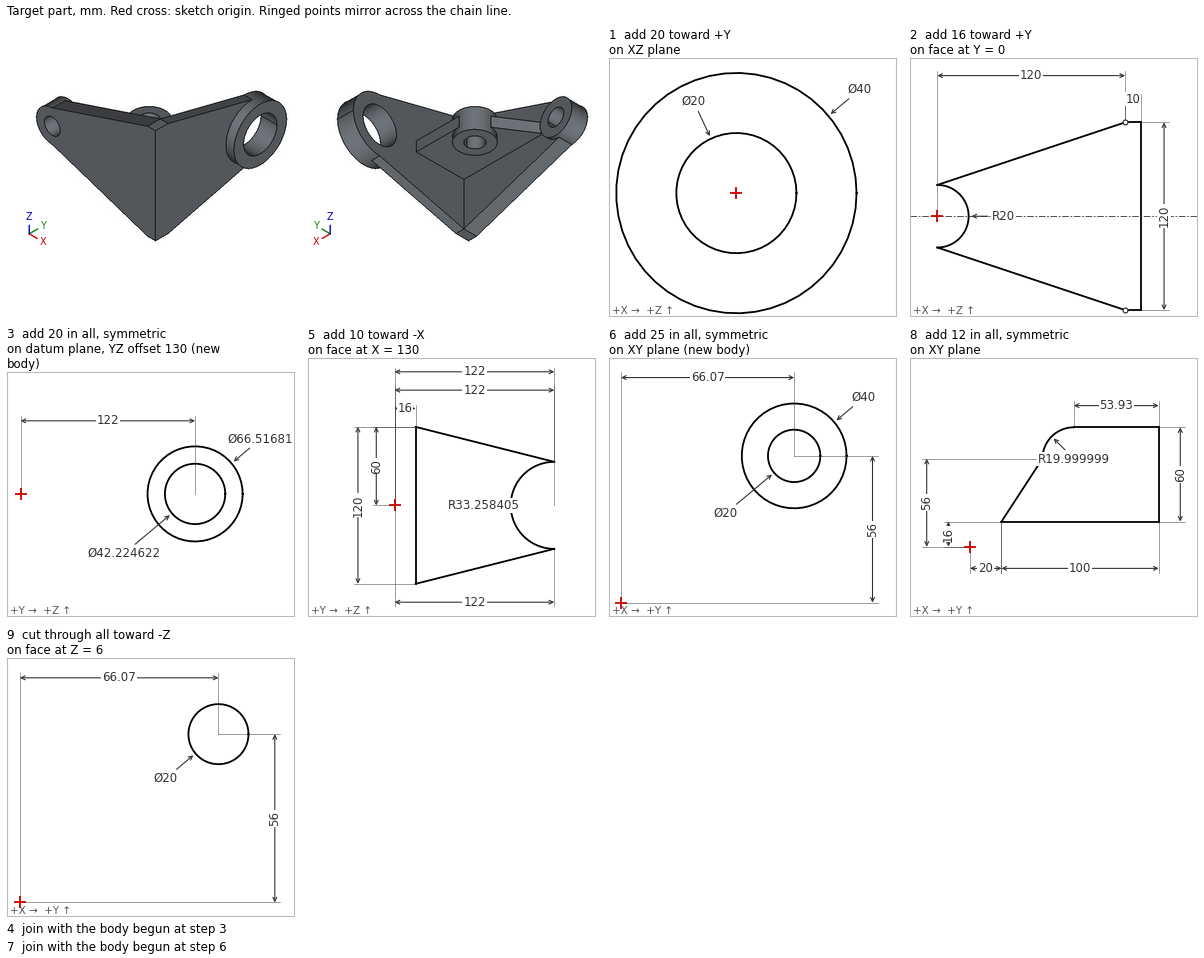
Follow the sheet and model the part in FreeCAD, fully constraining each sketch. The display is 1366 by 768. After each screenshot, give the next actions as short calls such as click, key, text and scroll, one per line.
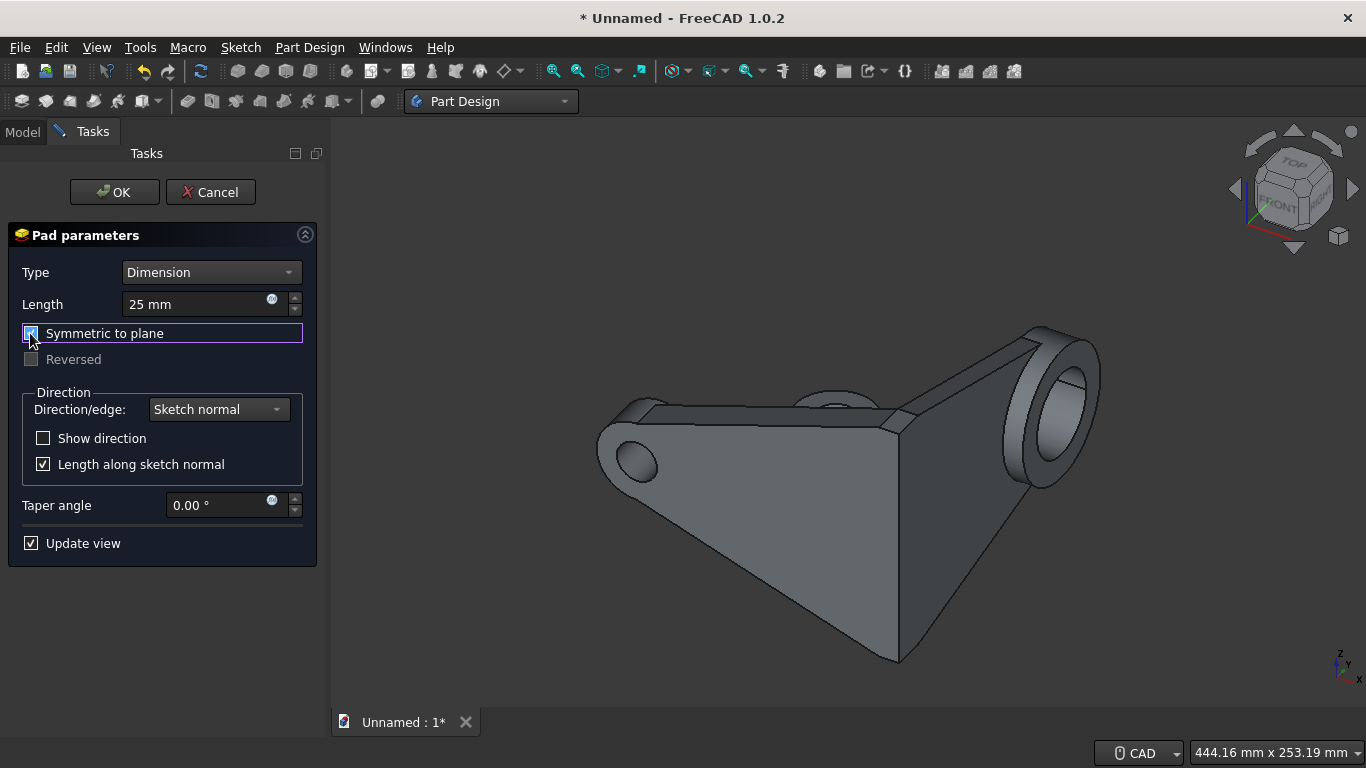
click(115, 192)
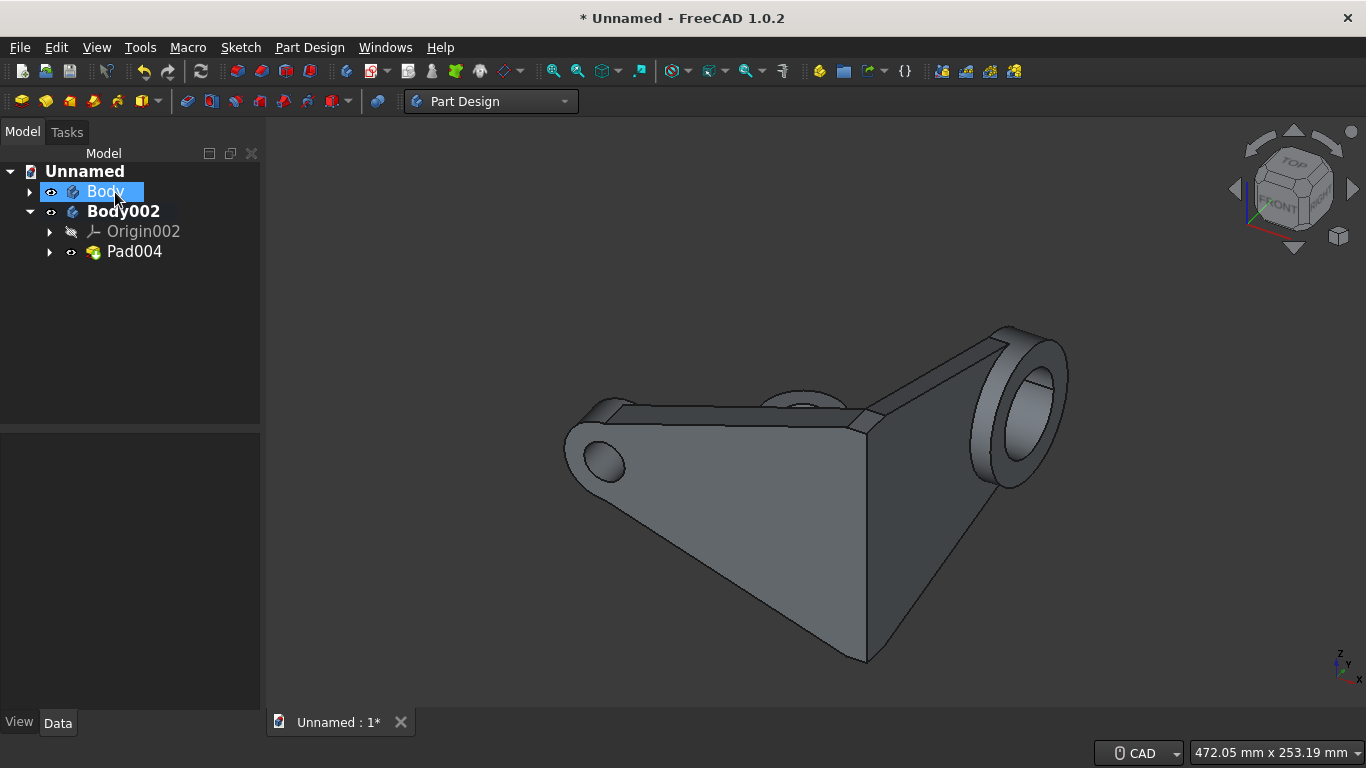
click(554, 72)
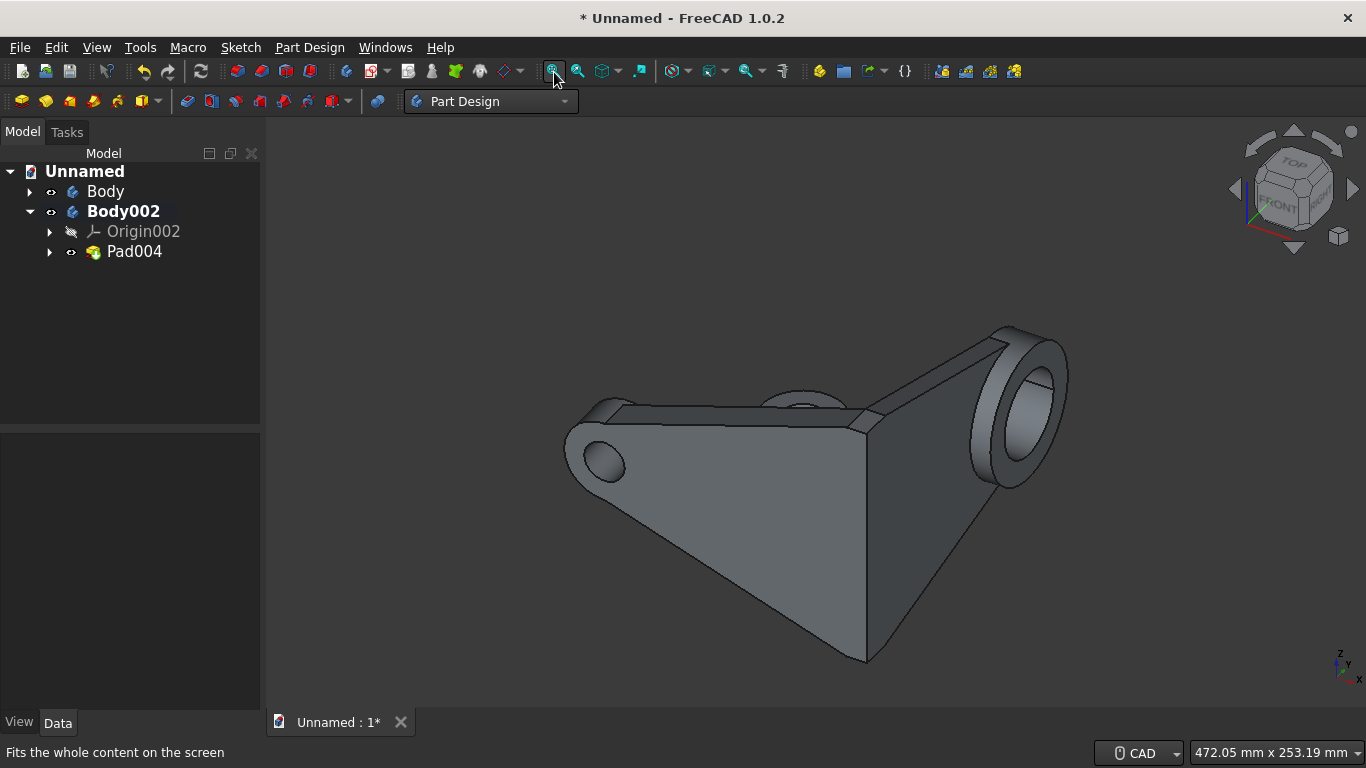
double_click(96, 192)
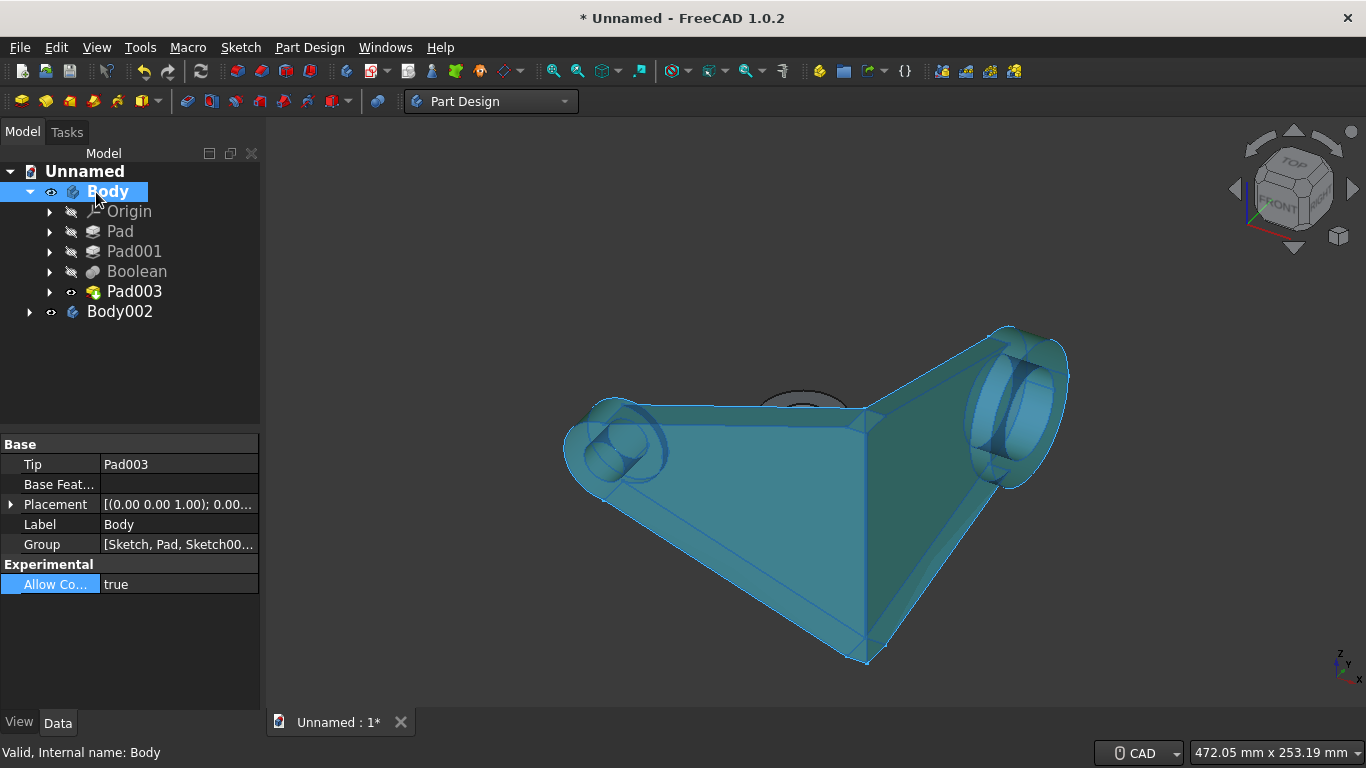
click(96, 312)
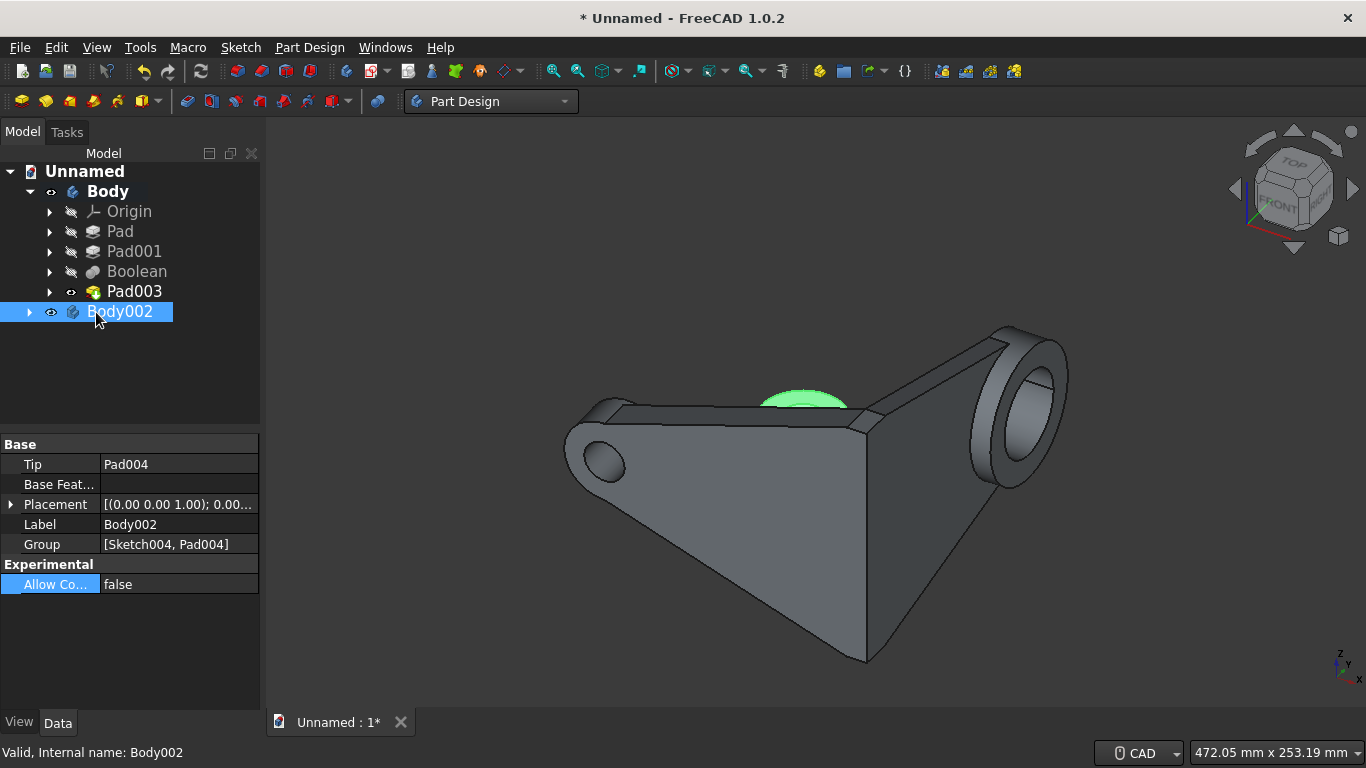
click(378, 102)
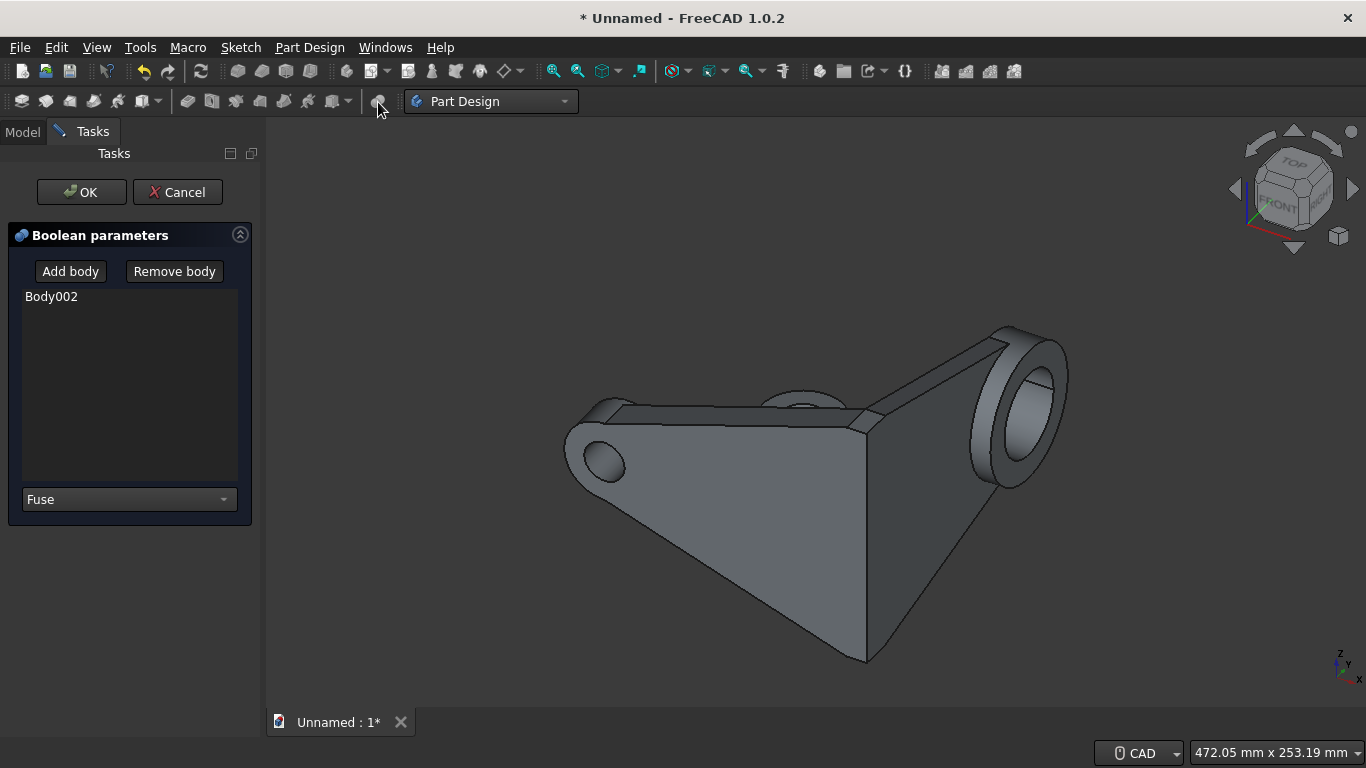
click(82, 192)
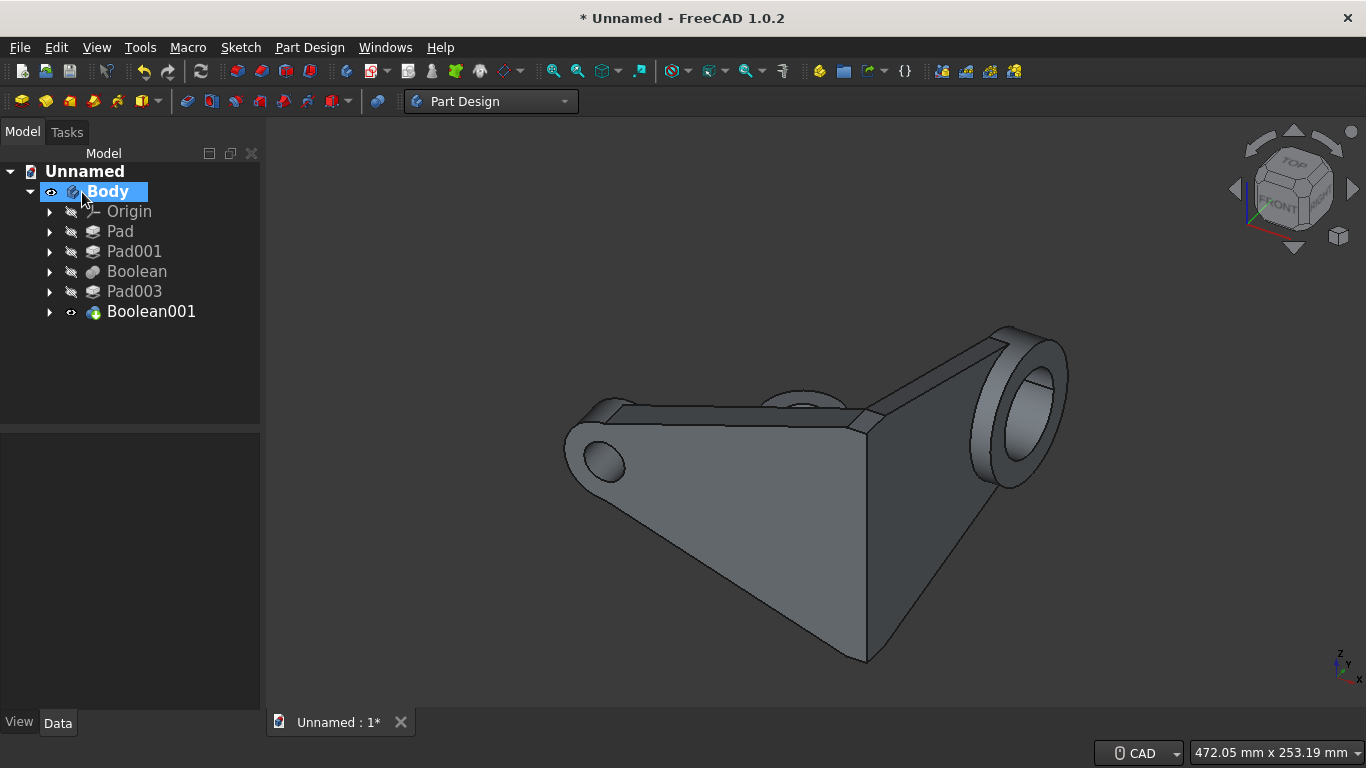
click(372, 72)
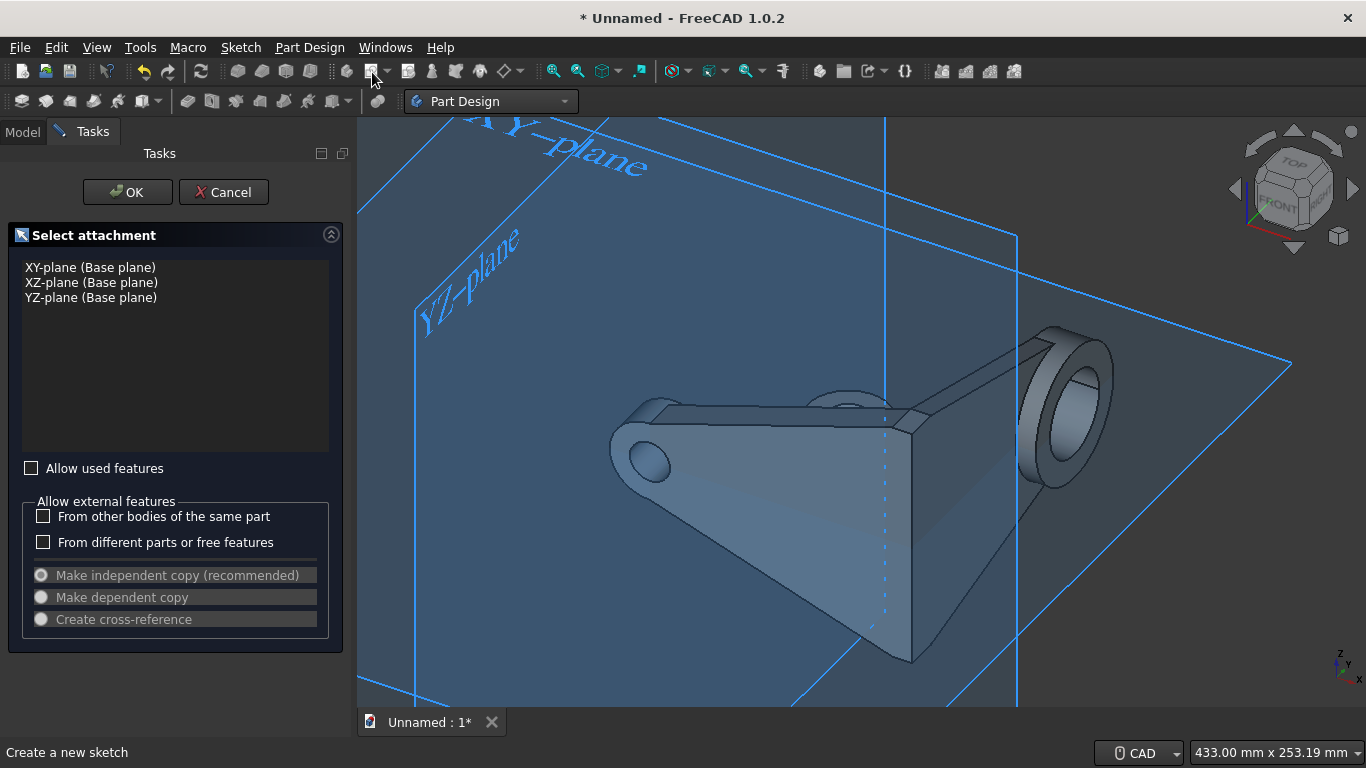
click(82, 268)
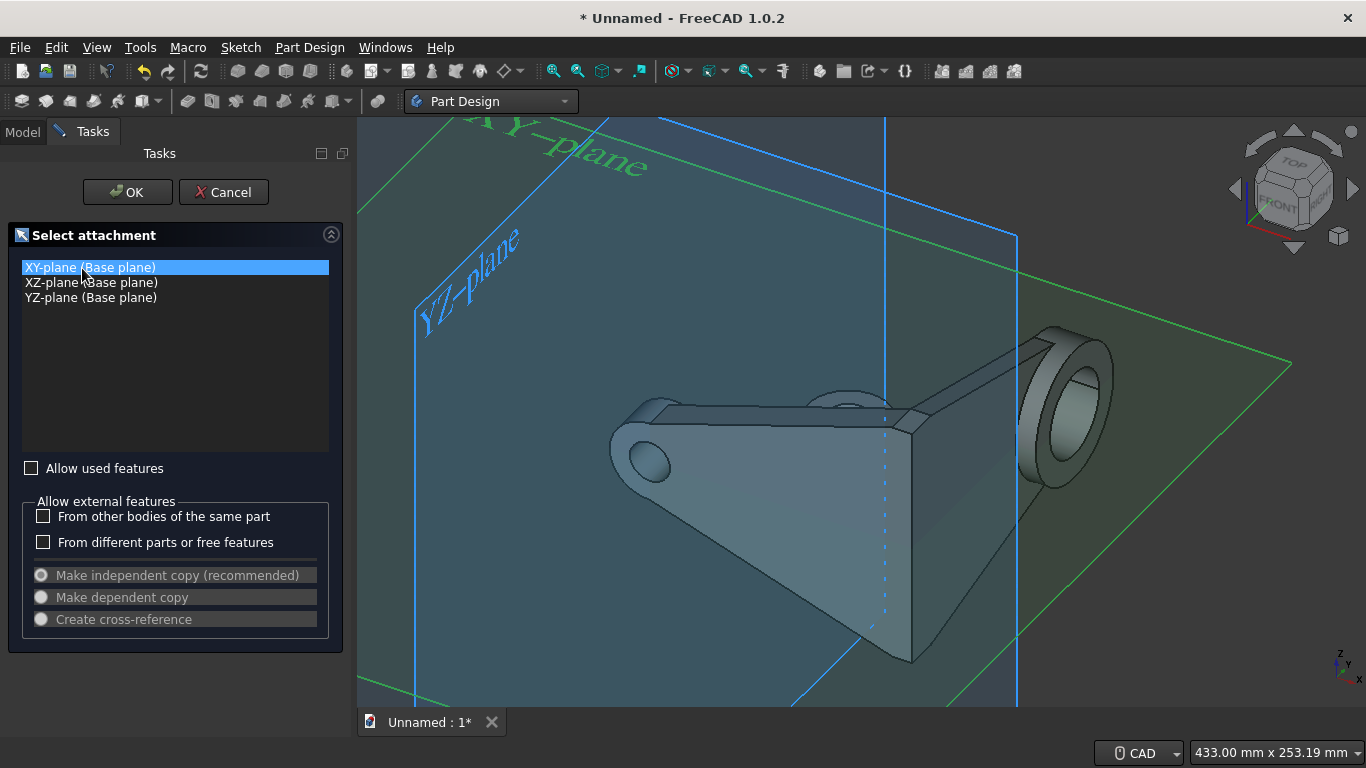
click(128, 192)